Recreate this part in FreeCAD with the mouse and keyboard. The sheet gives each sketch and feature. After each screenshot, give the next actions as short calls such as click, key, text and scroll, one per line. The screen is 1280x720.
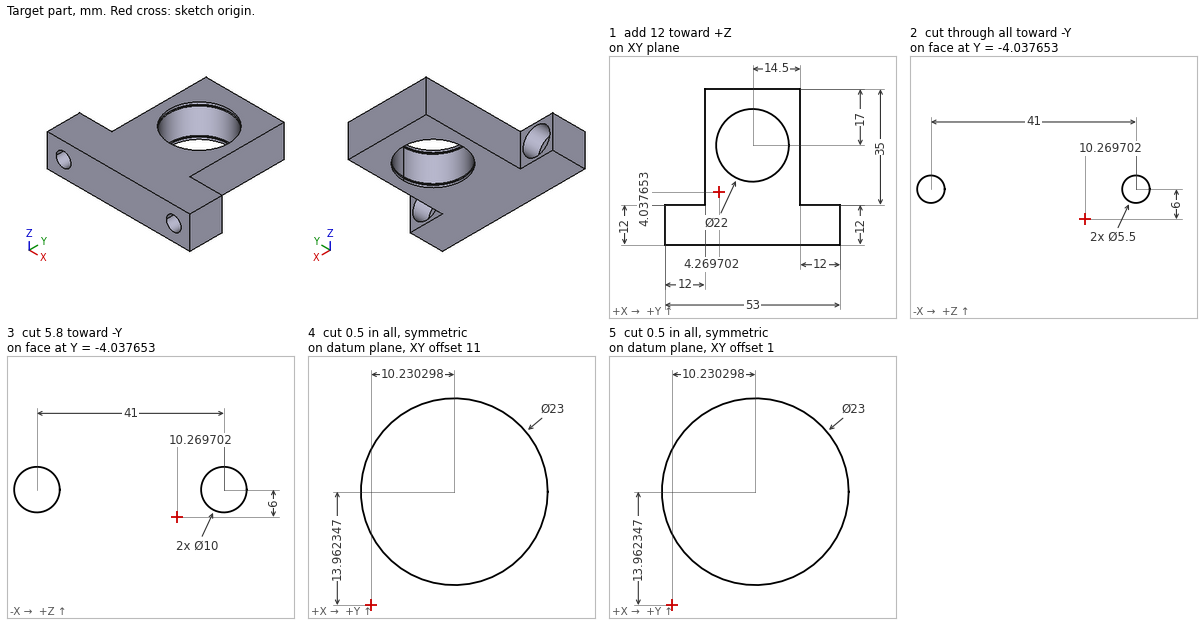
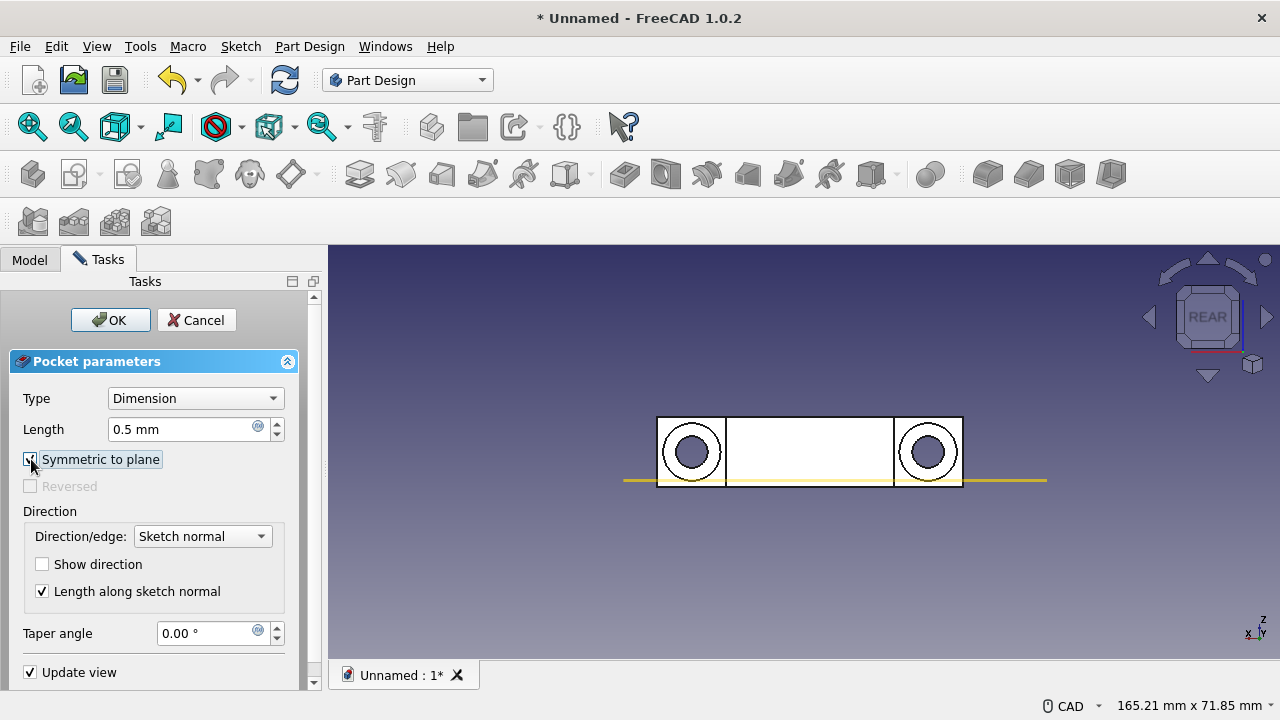
click(111, 320)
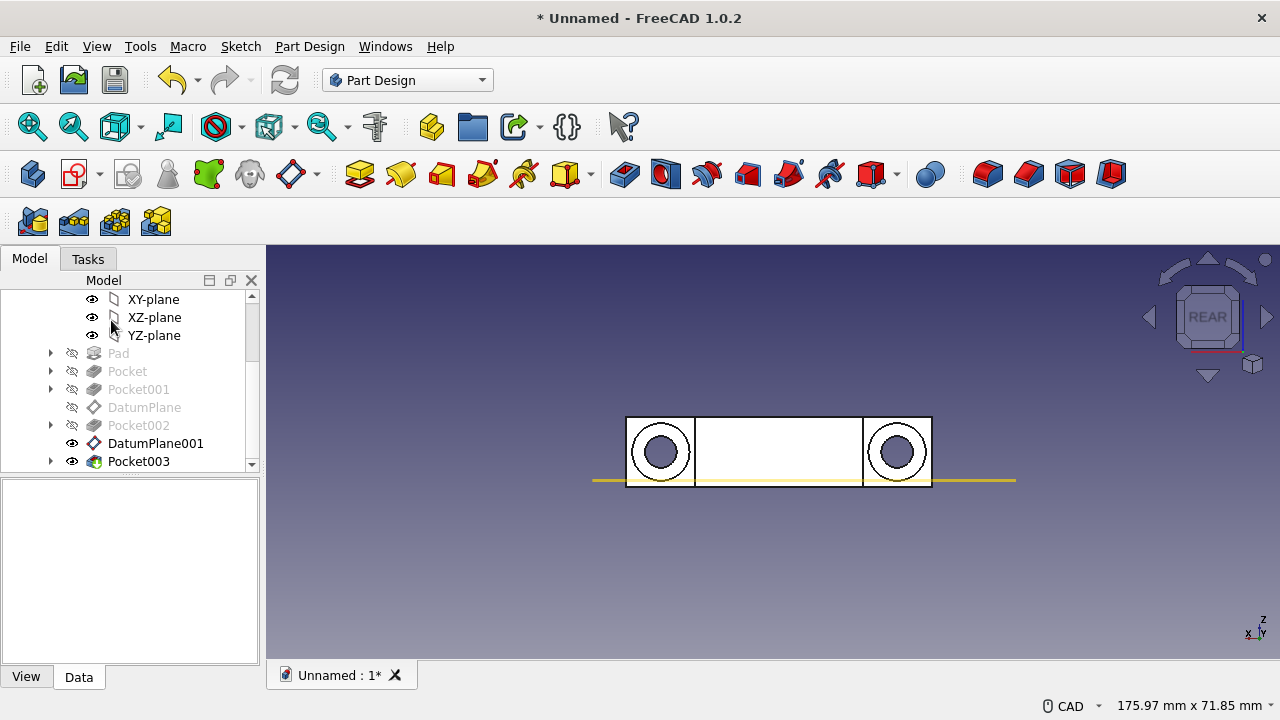
click(117, 443)
key(space)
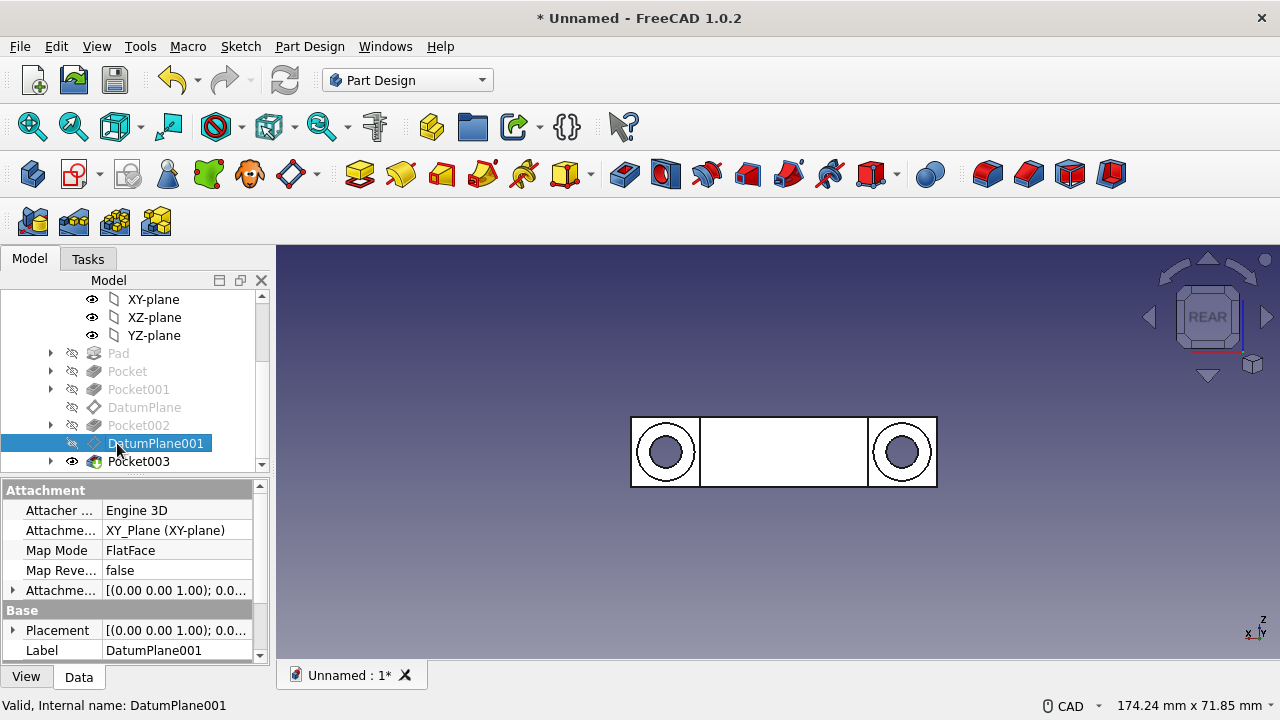
key(0)